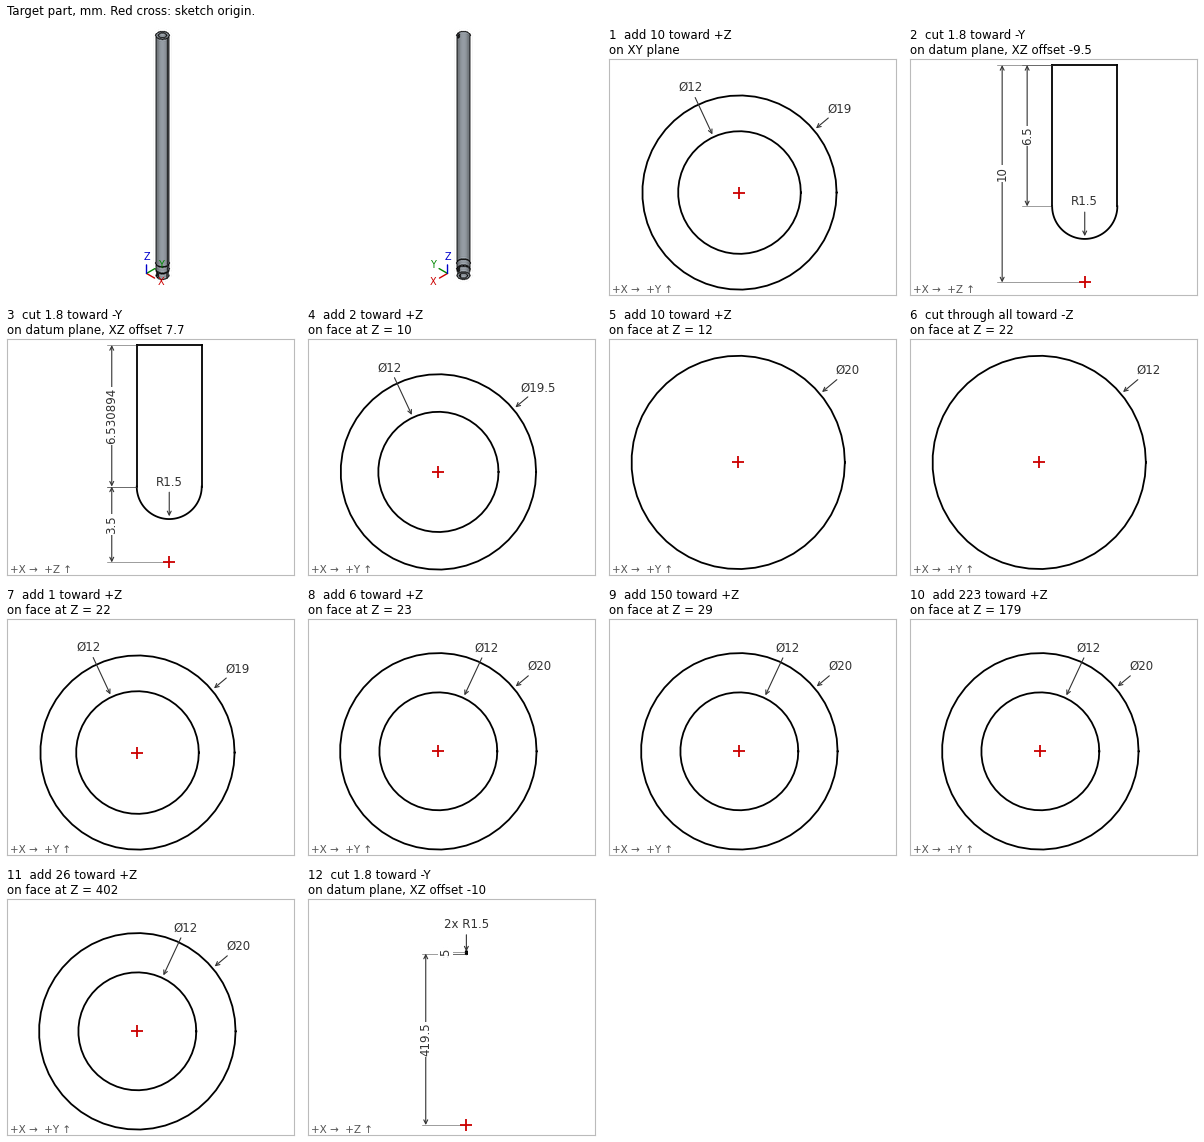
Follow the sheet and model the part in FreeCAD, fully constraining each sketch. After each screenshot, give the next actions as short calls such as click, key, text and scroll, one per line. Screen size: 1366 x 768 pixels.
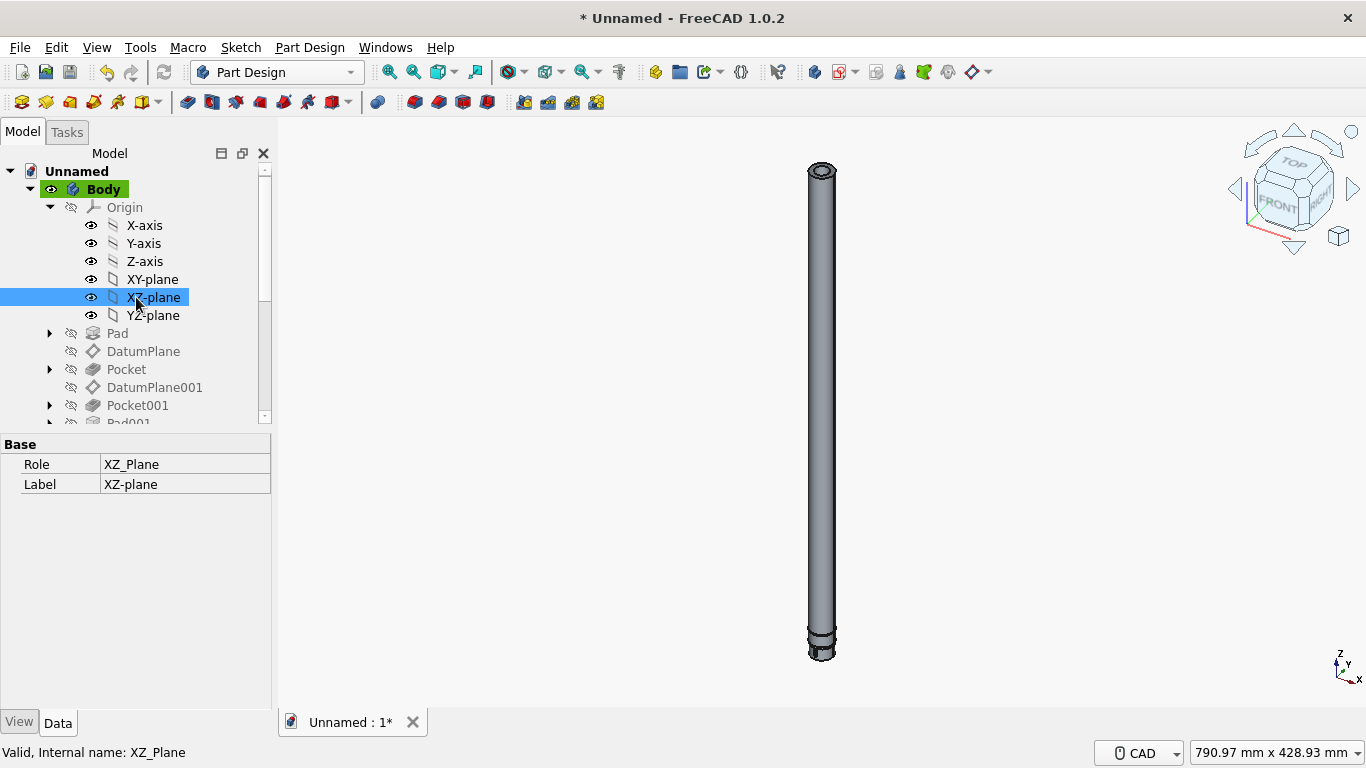
click(972, 72)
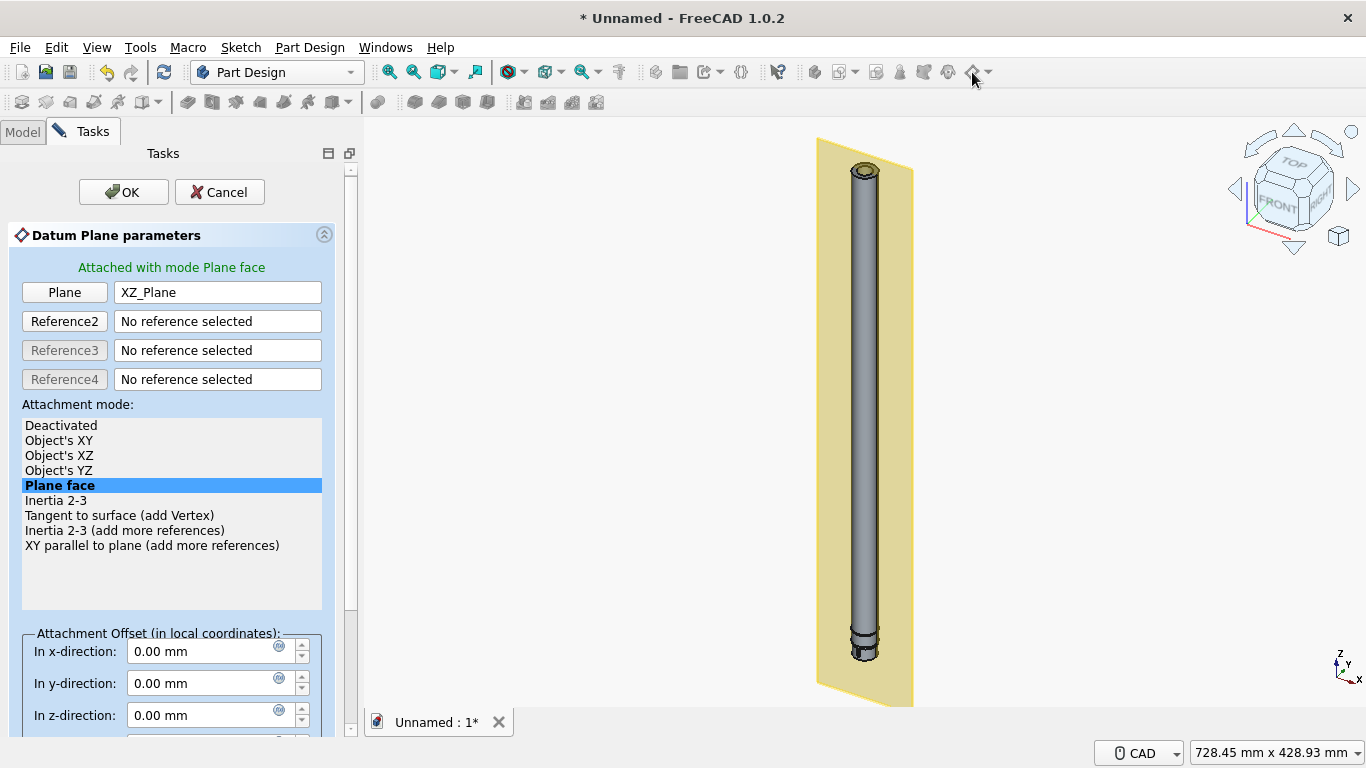
triple_click(210, 715)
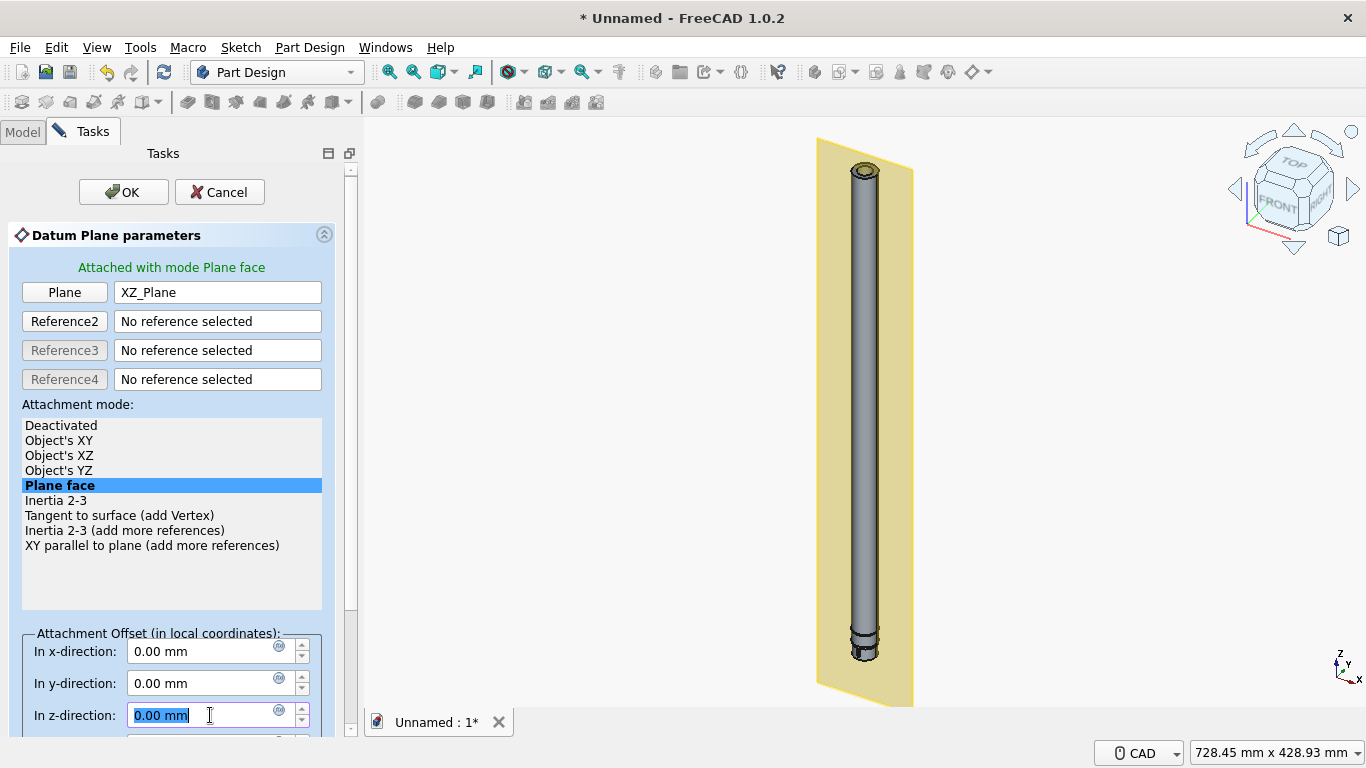
text(-10)
key(Tab)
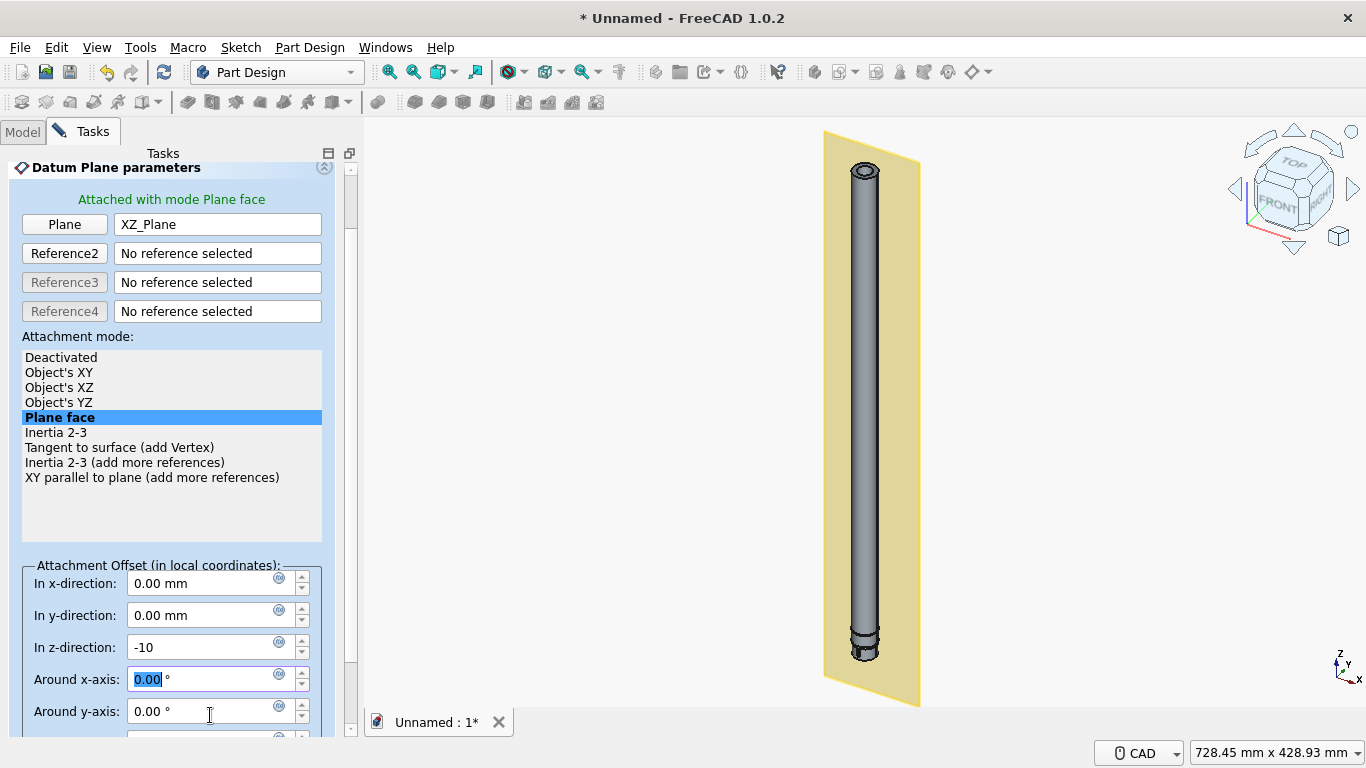
scroll(351, 450, up, 2)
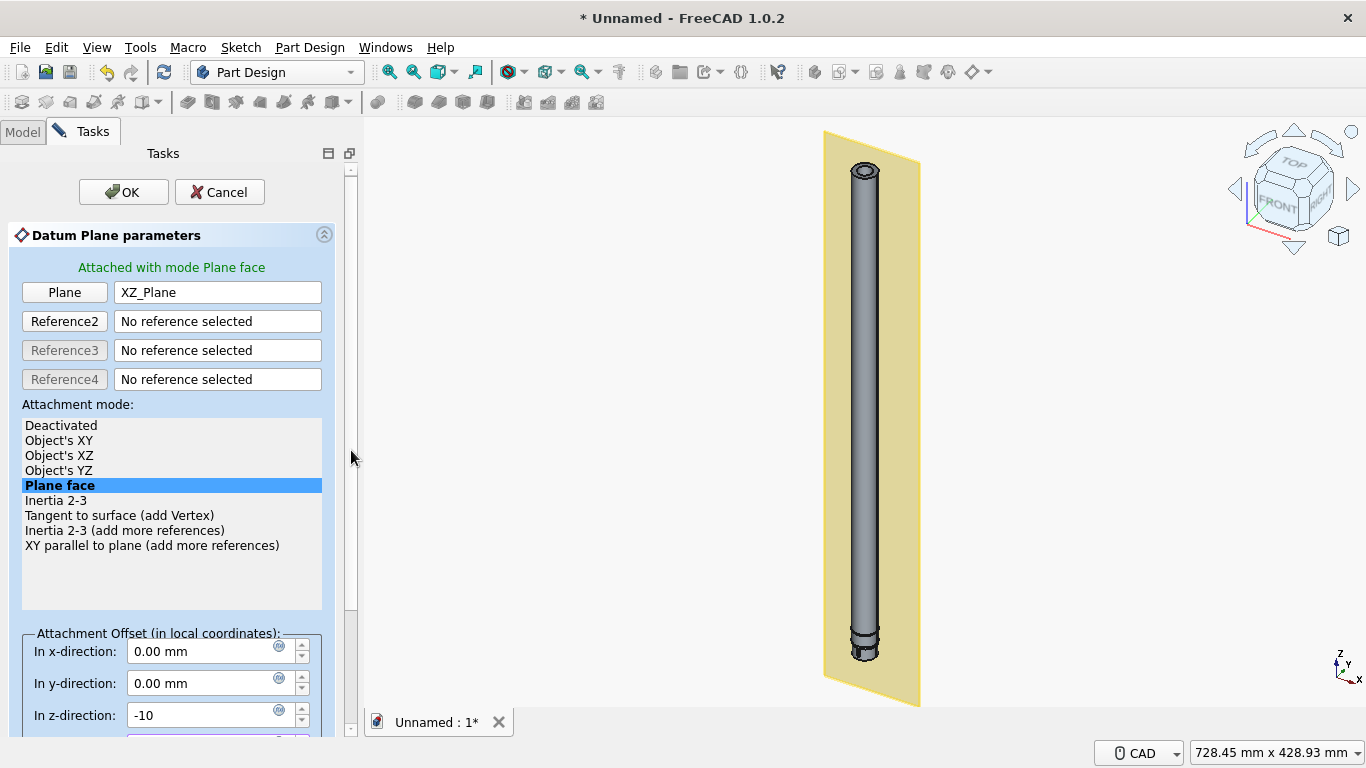
click(124, 192)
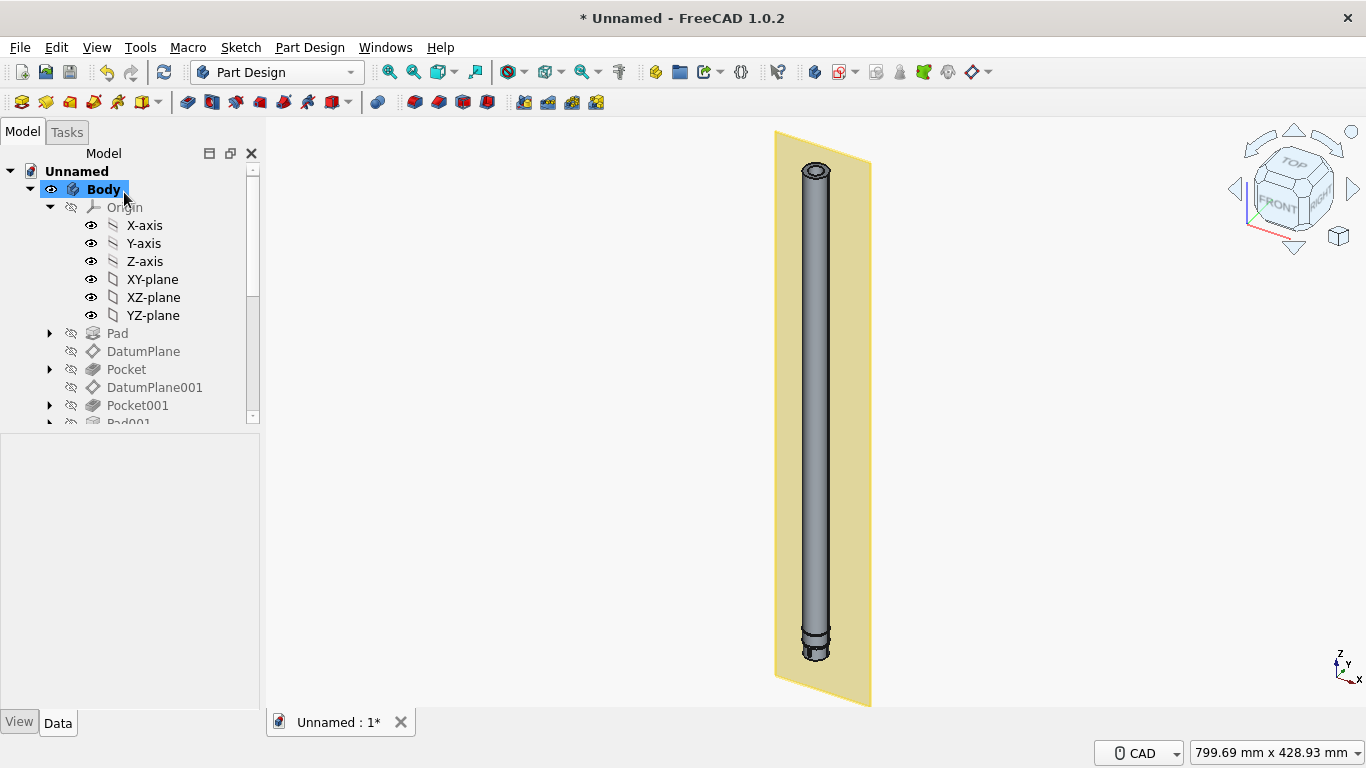
scroll(100, 293, down, 3)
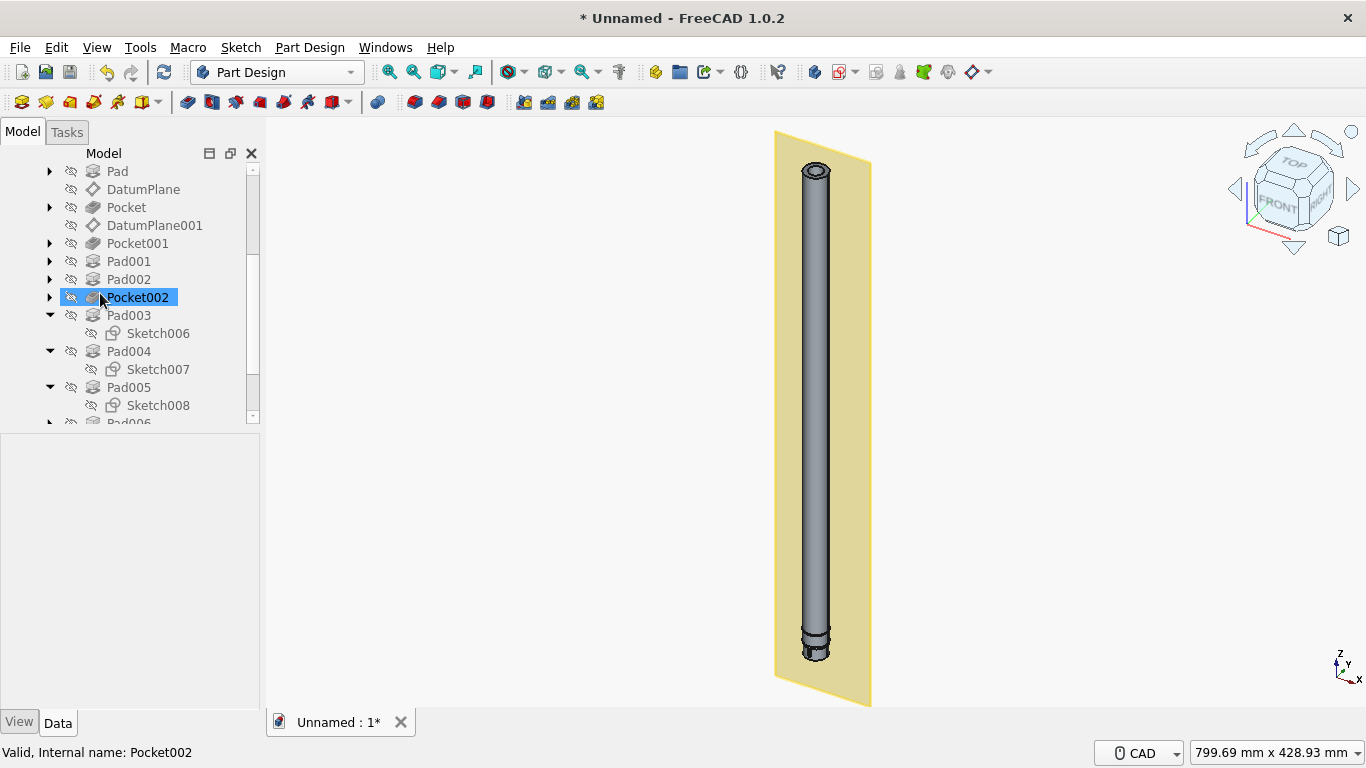
scroll(140, 293, up, 15)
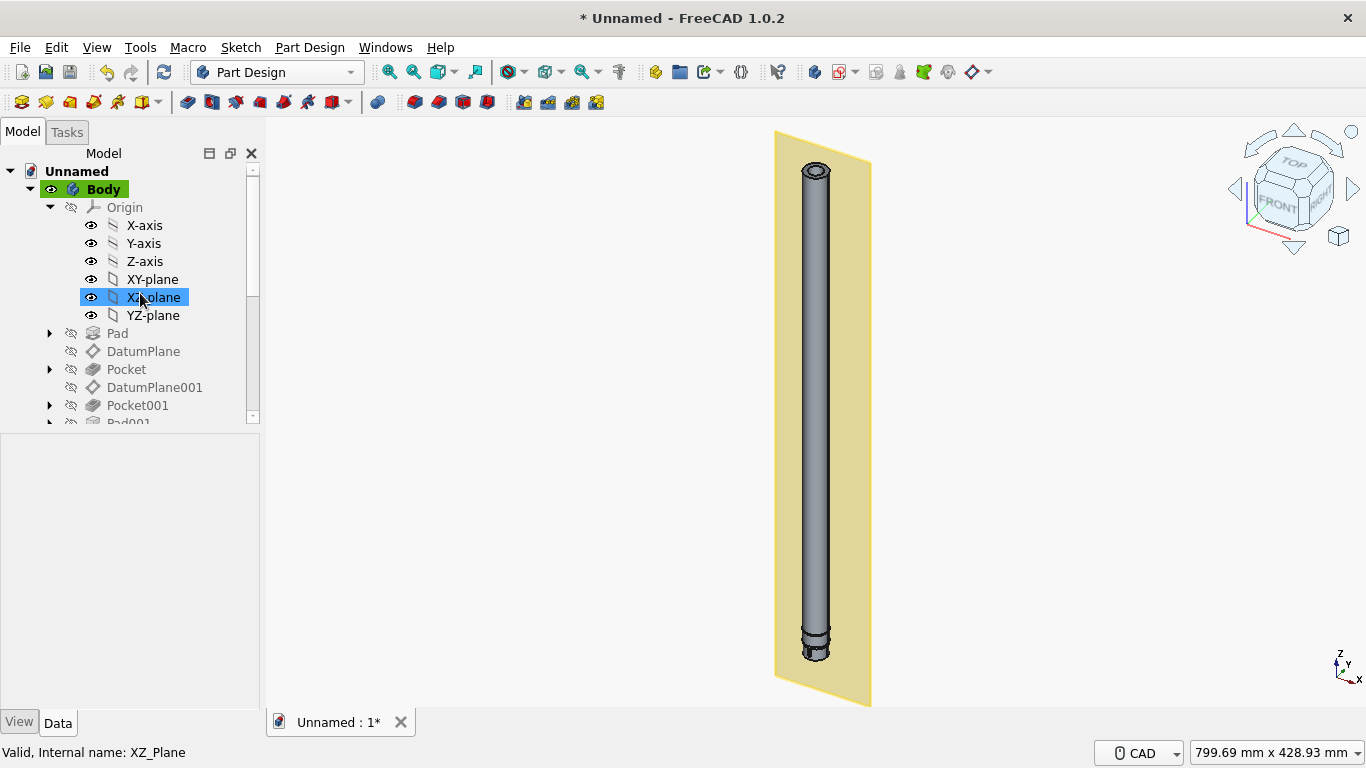
scroll(100, 293, down, 6)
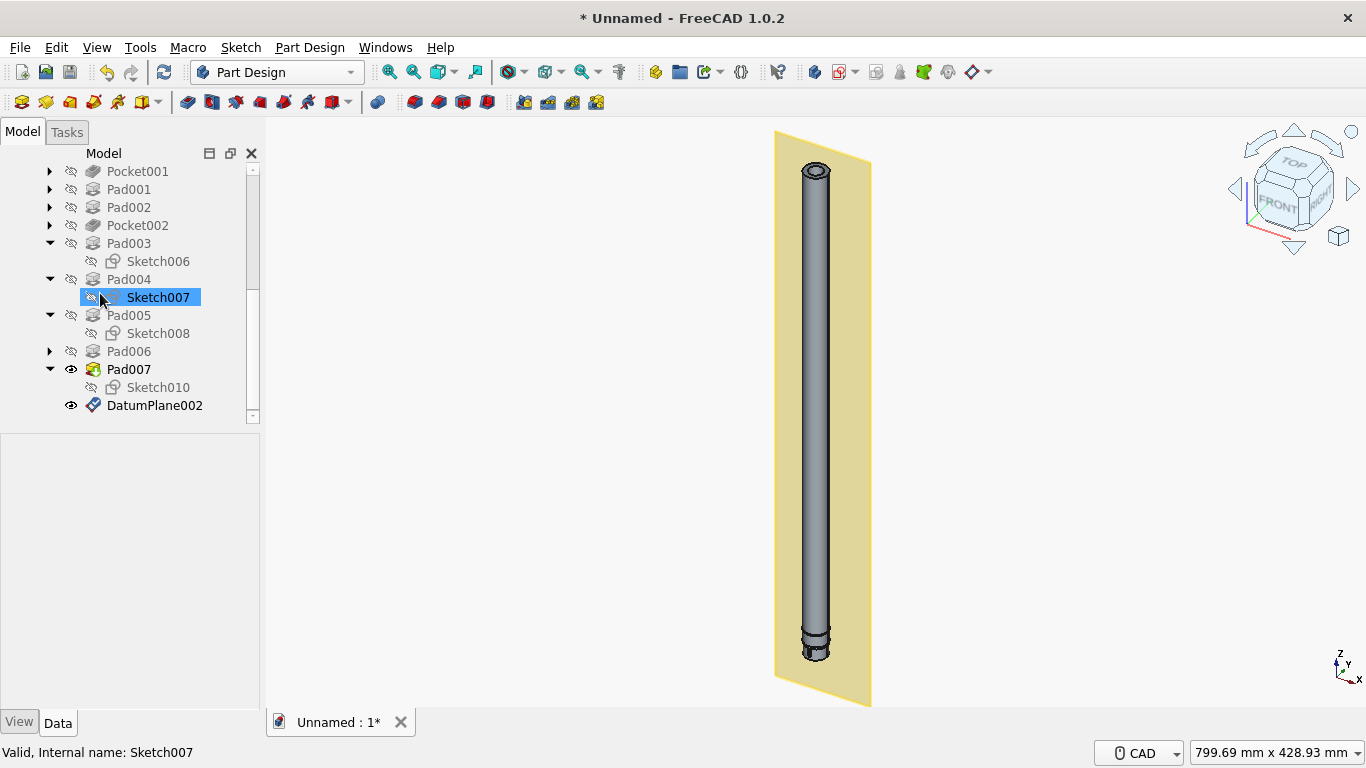
click(116, 405)